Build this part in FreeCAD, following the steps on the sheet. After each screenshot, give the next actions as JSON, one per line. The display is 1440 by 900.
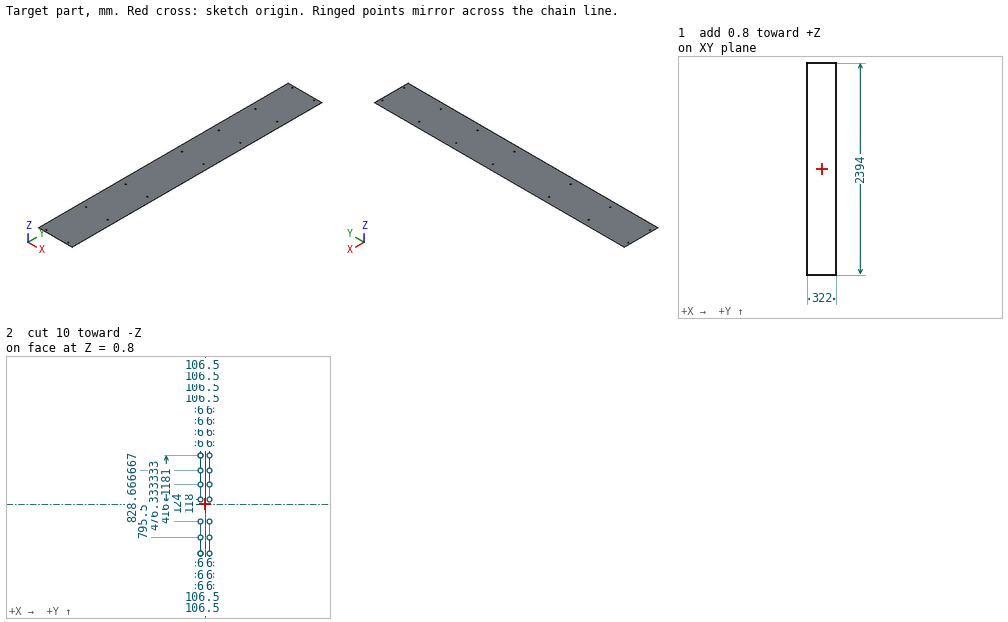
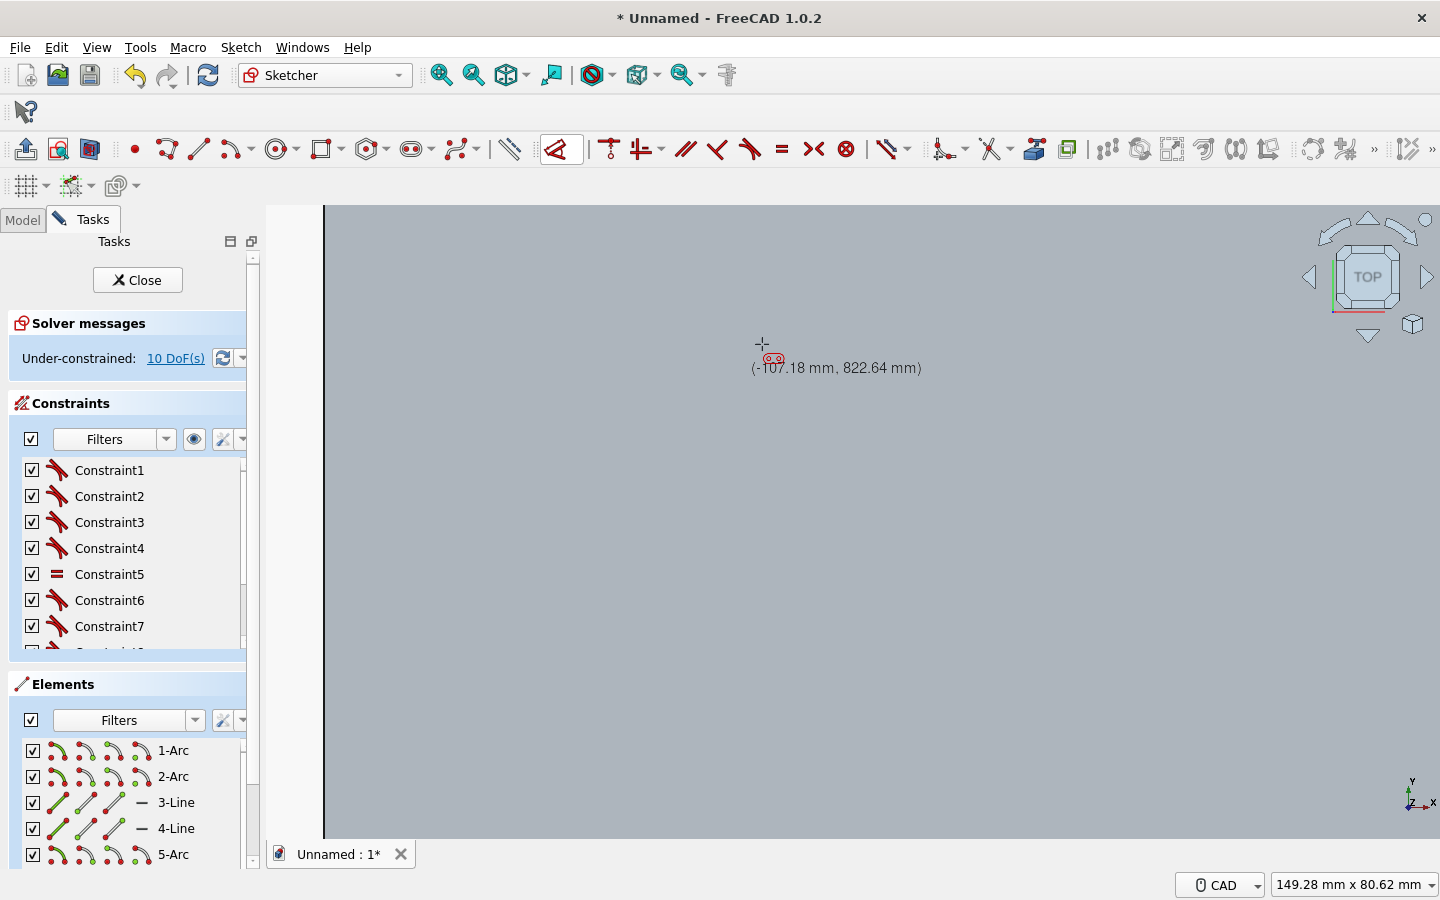
{"action": "scroll", "coordinate": [762, 344], "scroll_direction": "down", "scroll_amount": 18}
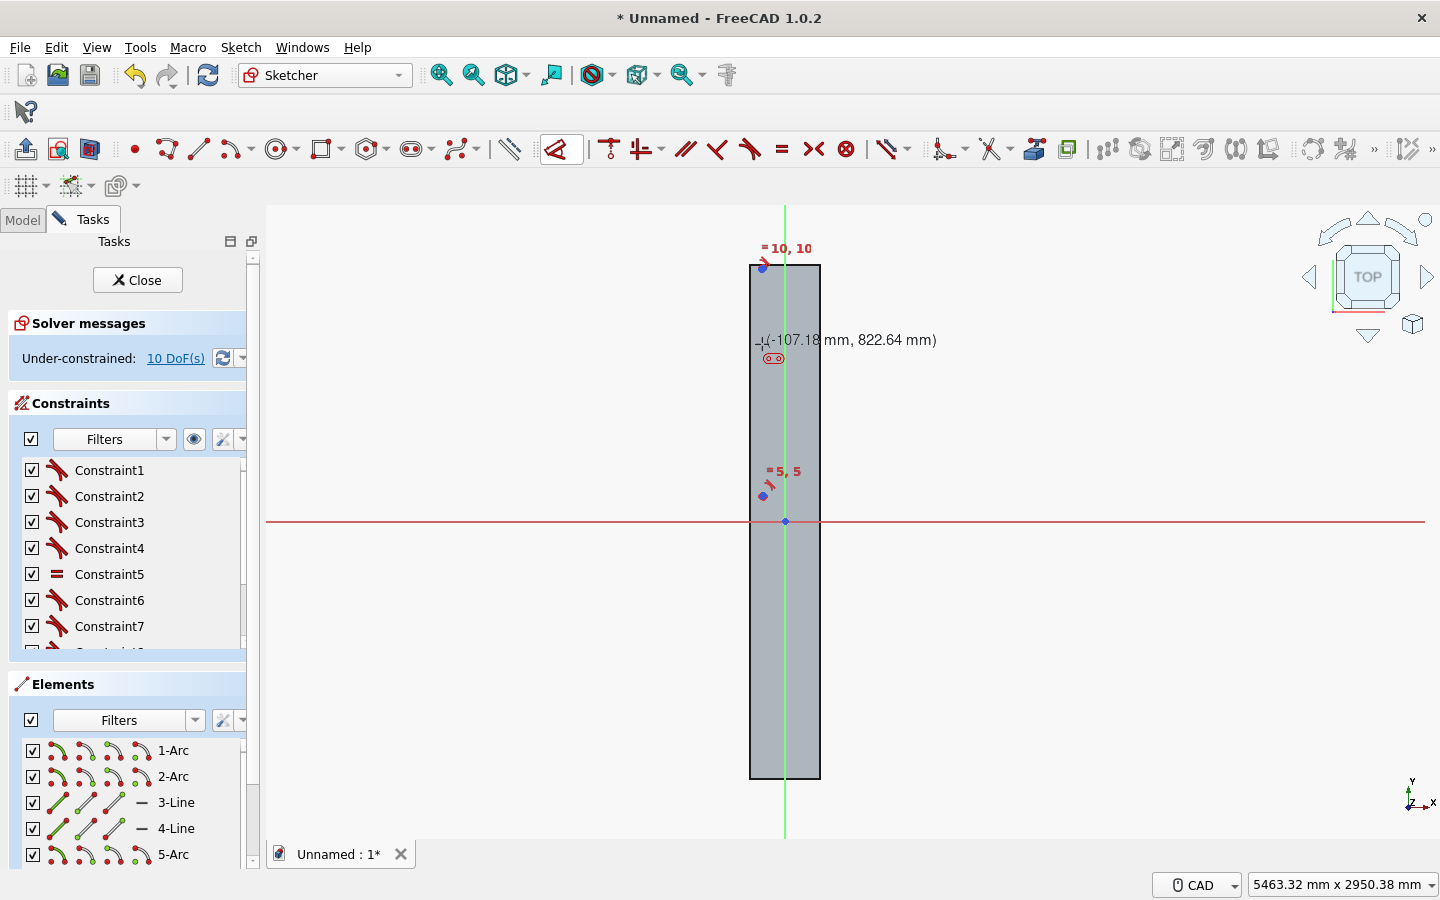
{"action": "left_click", "coordinate": [762, 344]}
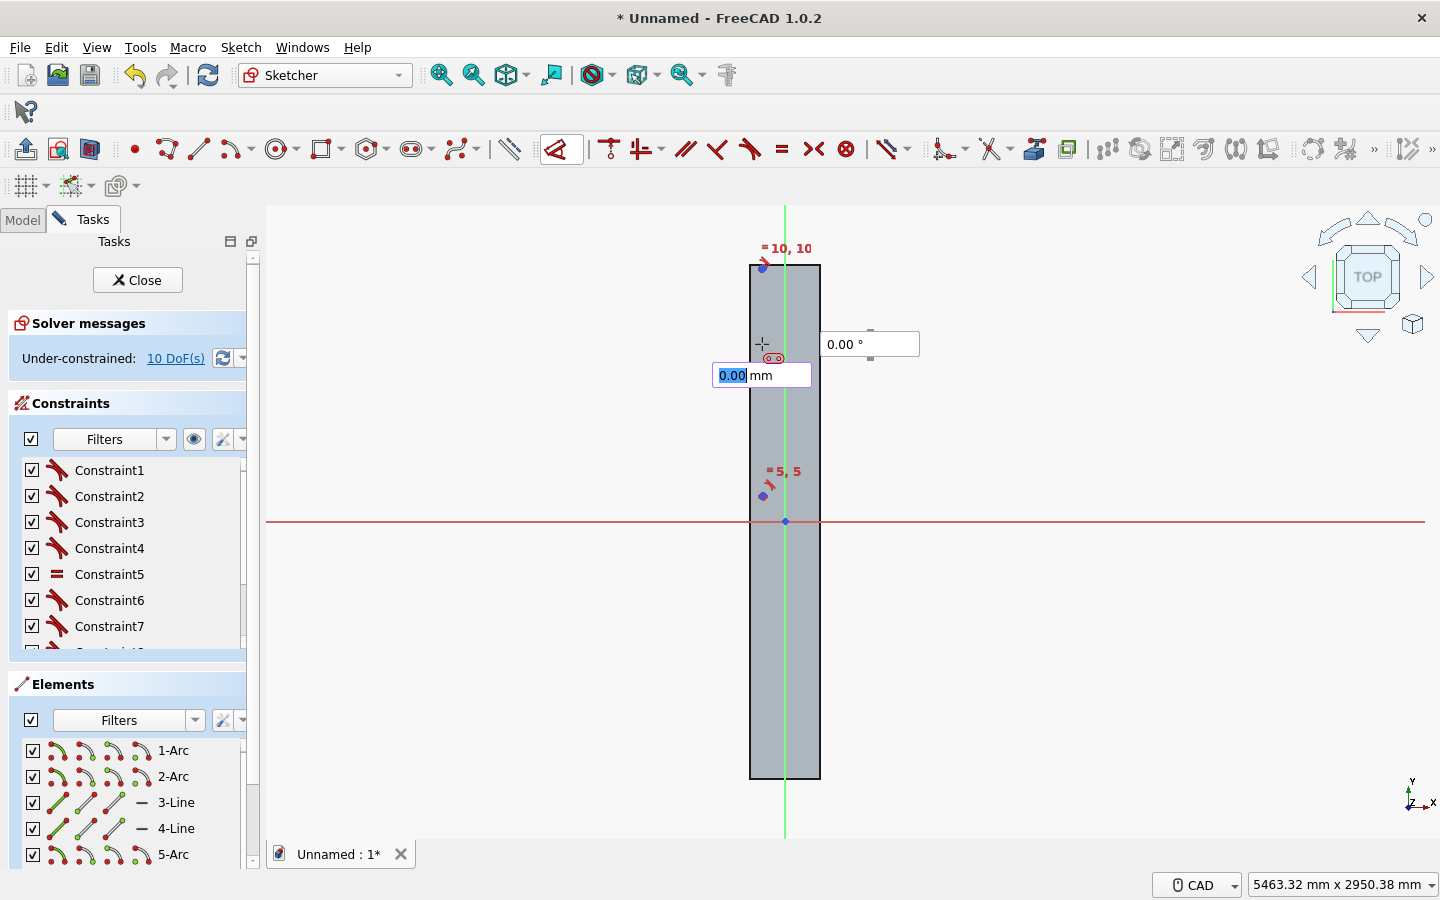
{"action": "scroll", "coordinate": [763, 344], "scroll_direction": "up", "scroll_amount": 13}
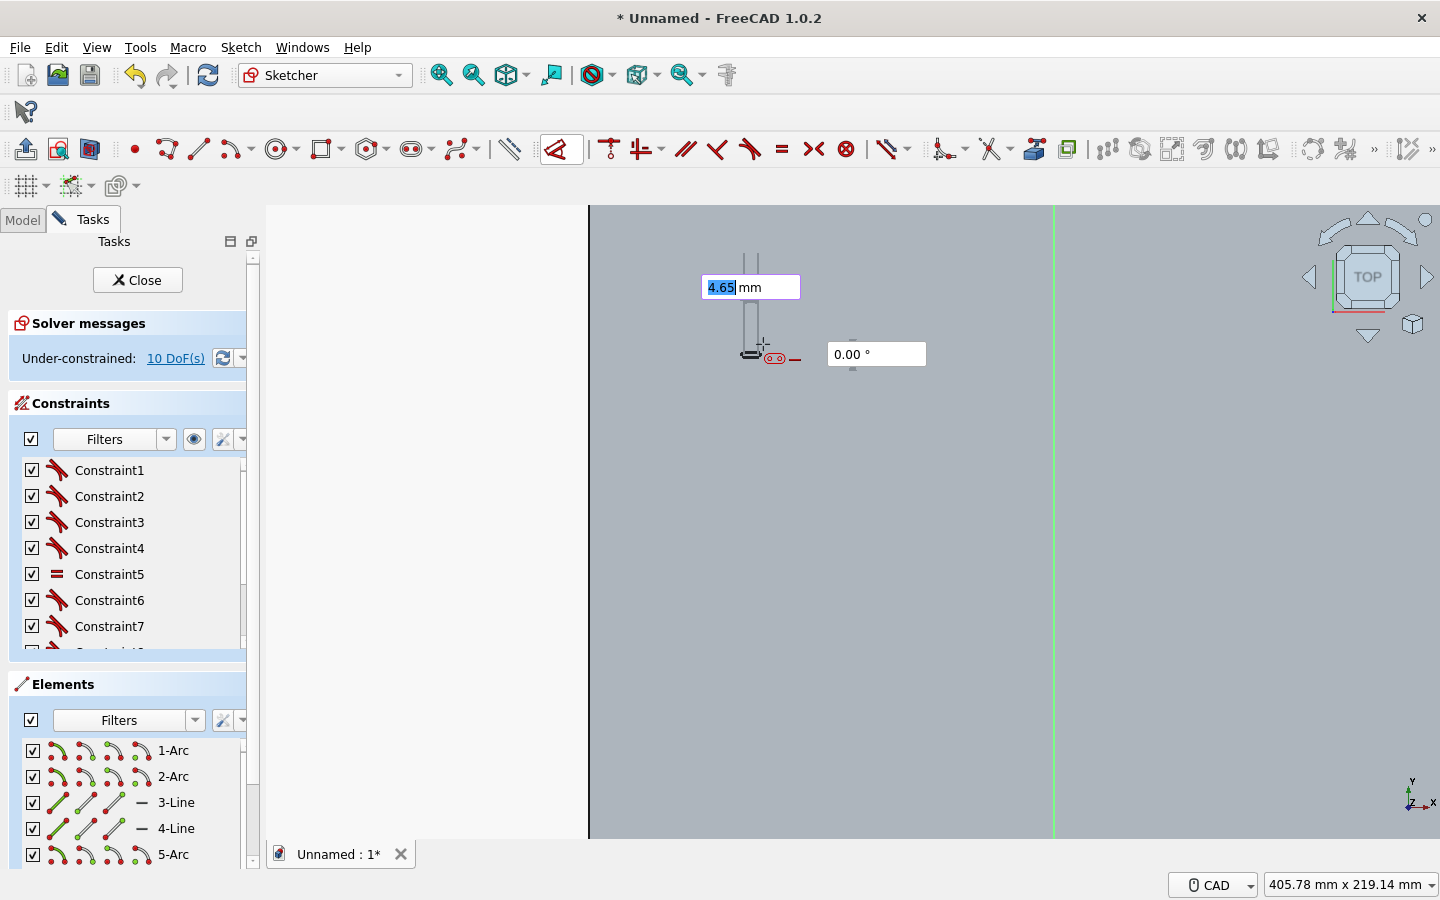
{"action": "left_click", "coordinate": [764, 341]}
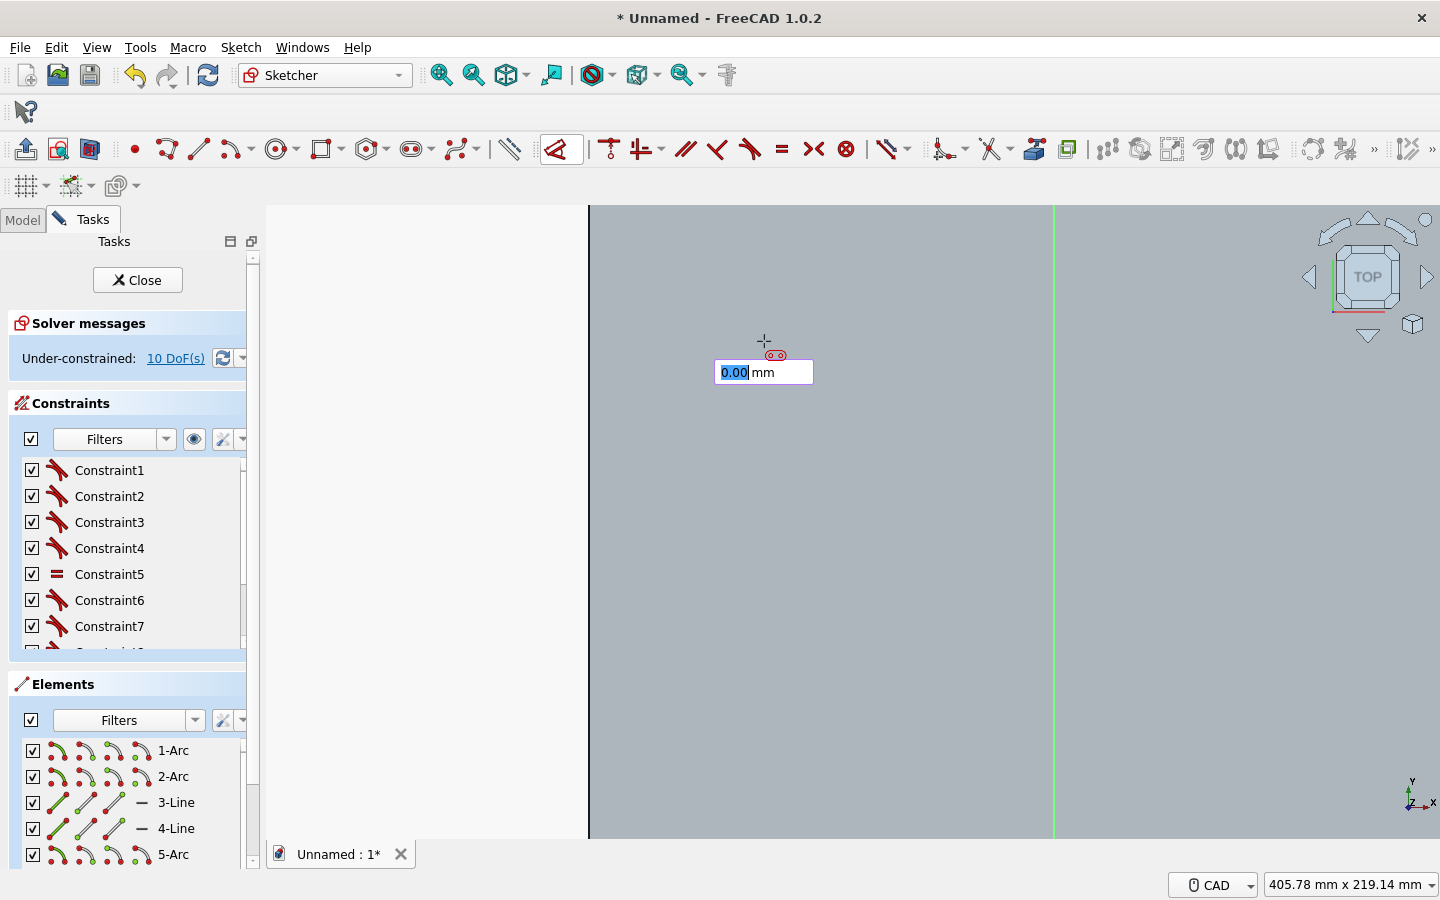
{"action": "scroll", "coordinate": [755, 337], "scroll_direction": "up", "scroll_amount": 4}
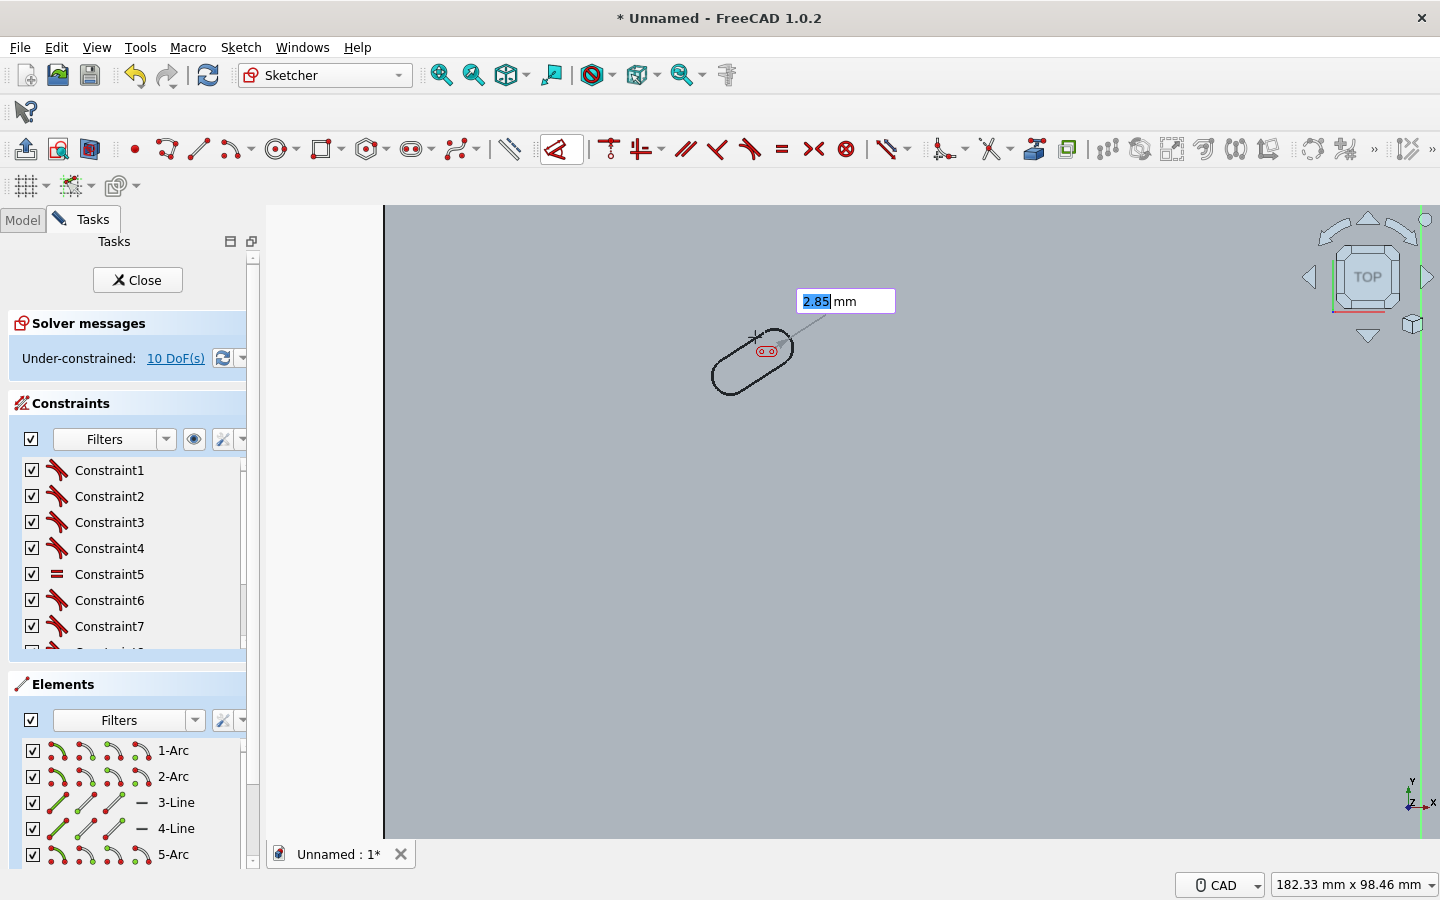
{"action": "left_click", "coordinate": [754, 337]}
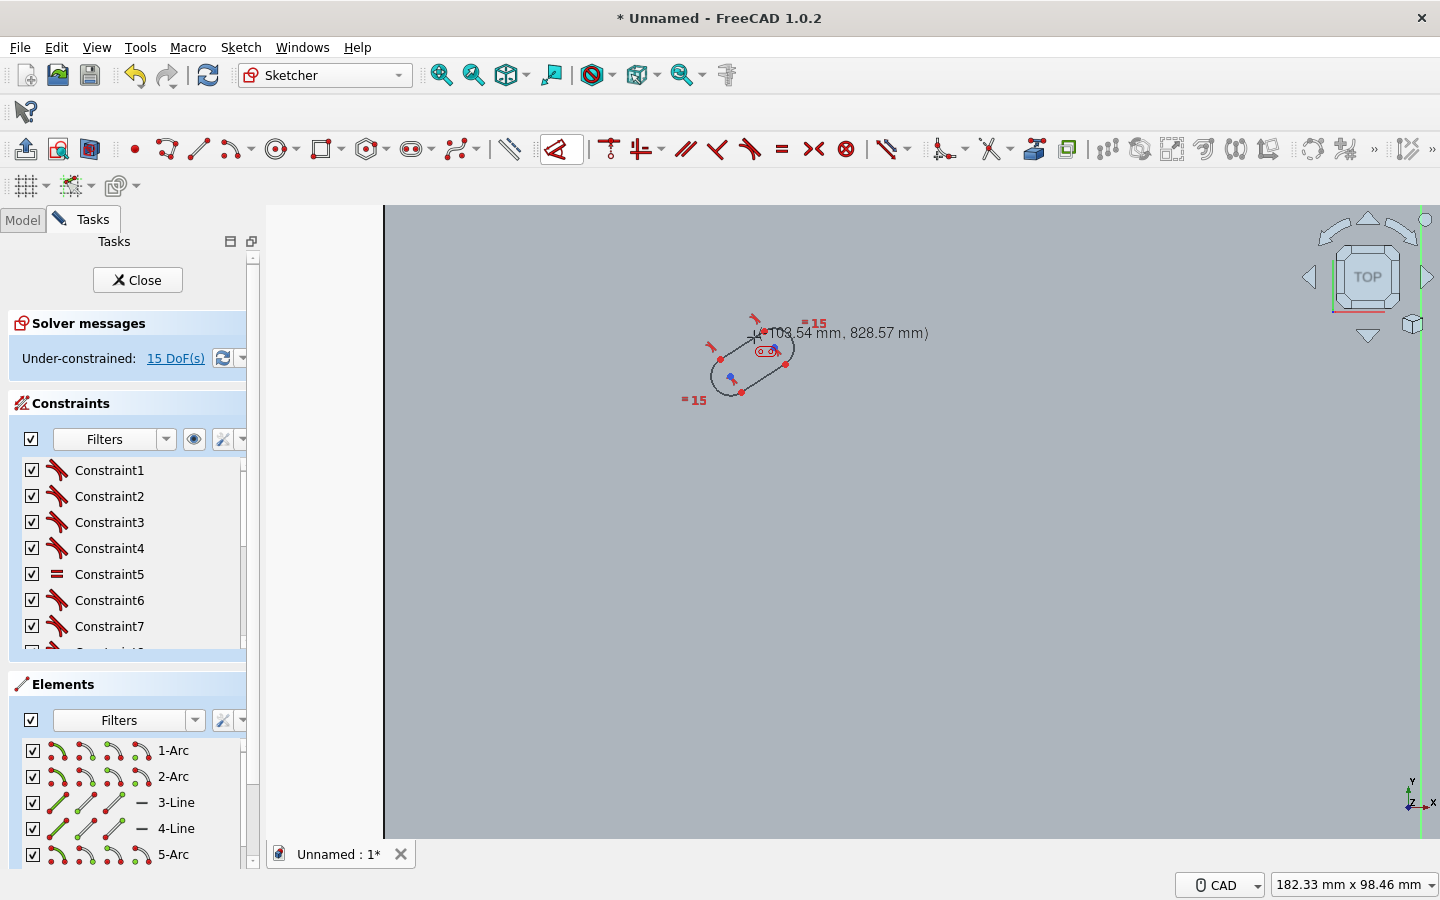
{"action": "scroll", "coordinate": [763, 344], "scroll_direction": "down", "scroll_amount": 17}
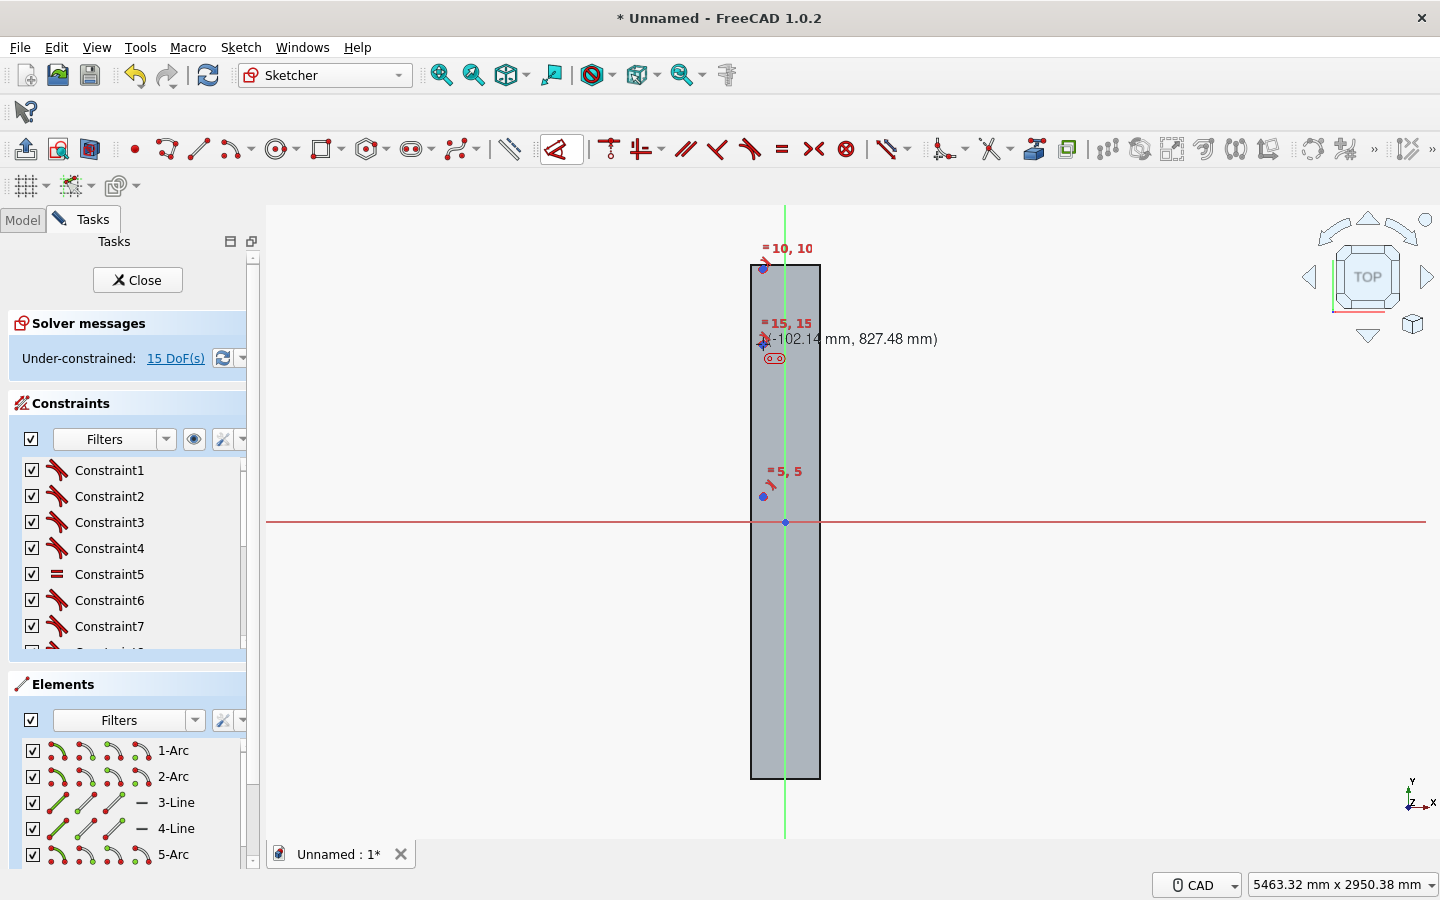
{"action": "scroll", "coordinate": [762, 775], "scroll_direction": "up", "scroll_amount": 18}